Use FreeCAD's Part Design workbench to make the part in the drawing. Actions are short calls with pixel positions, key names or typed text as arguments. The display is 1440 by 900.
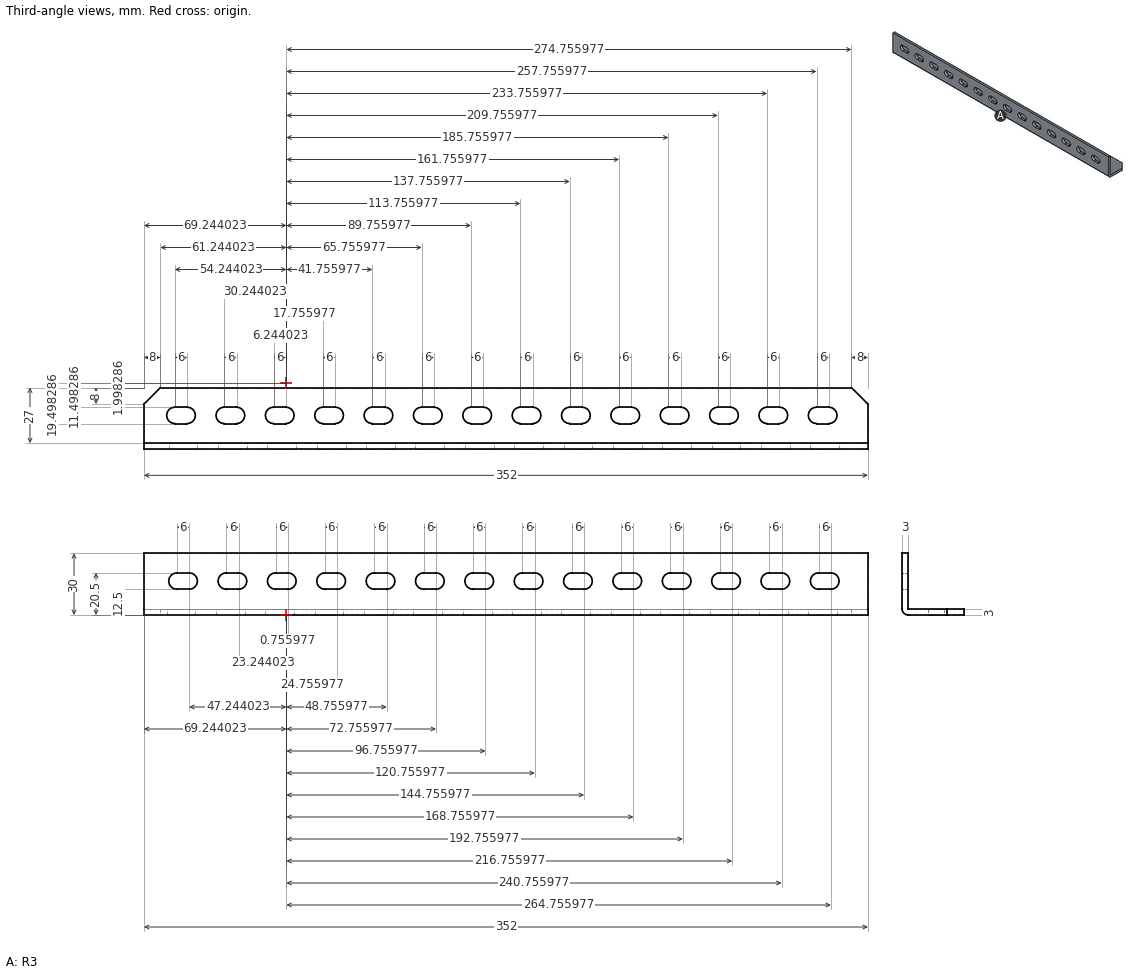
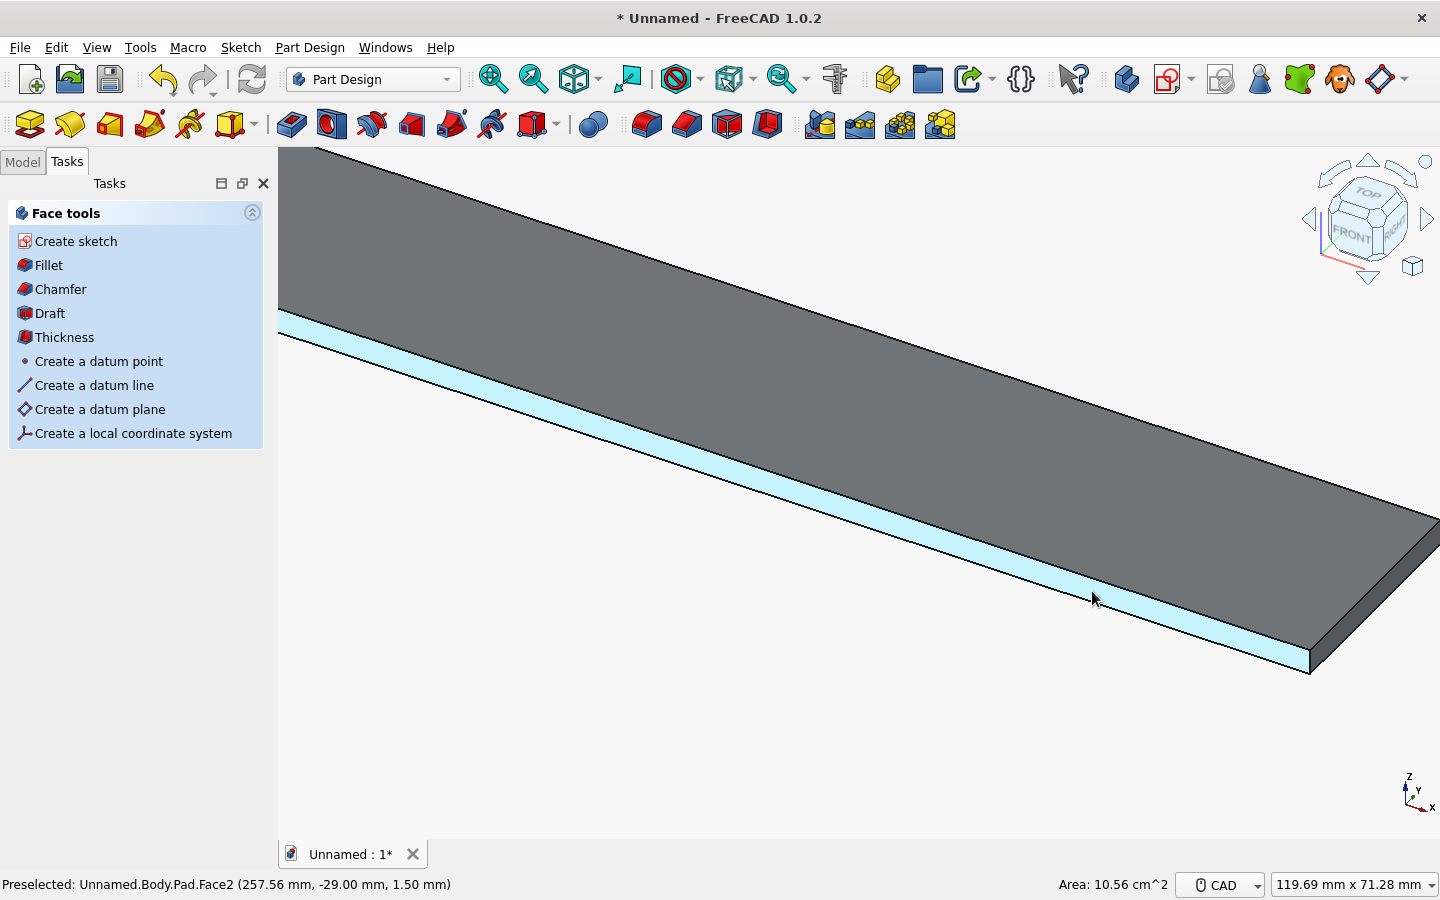
click(1168, 80)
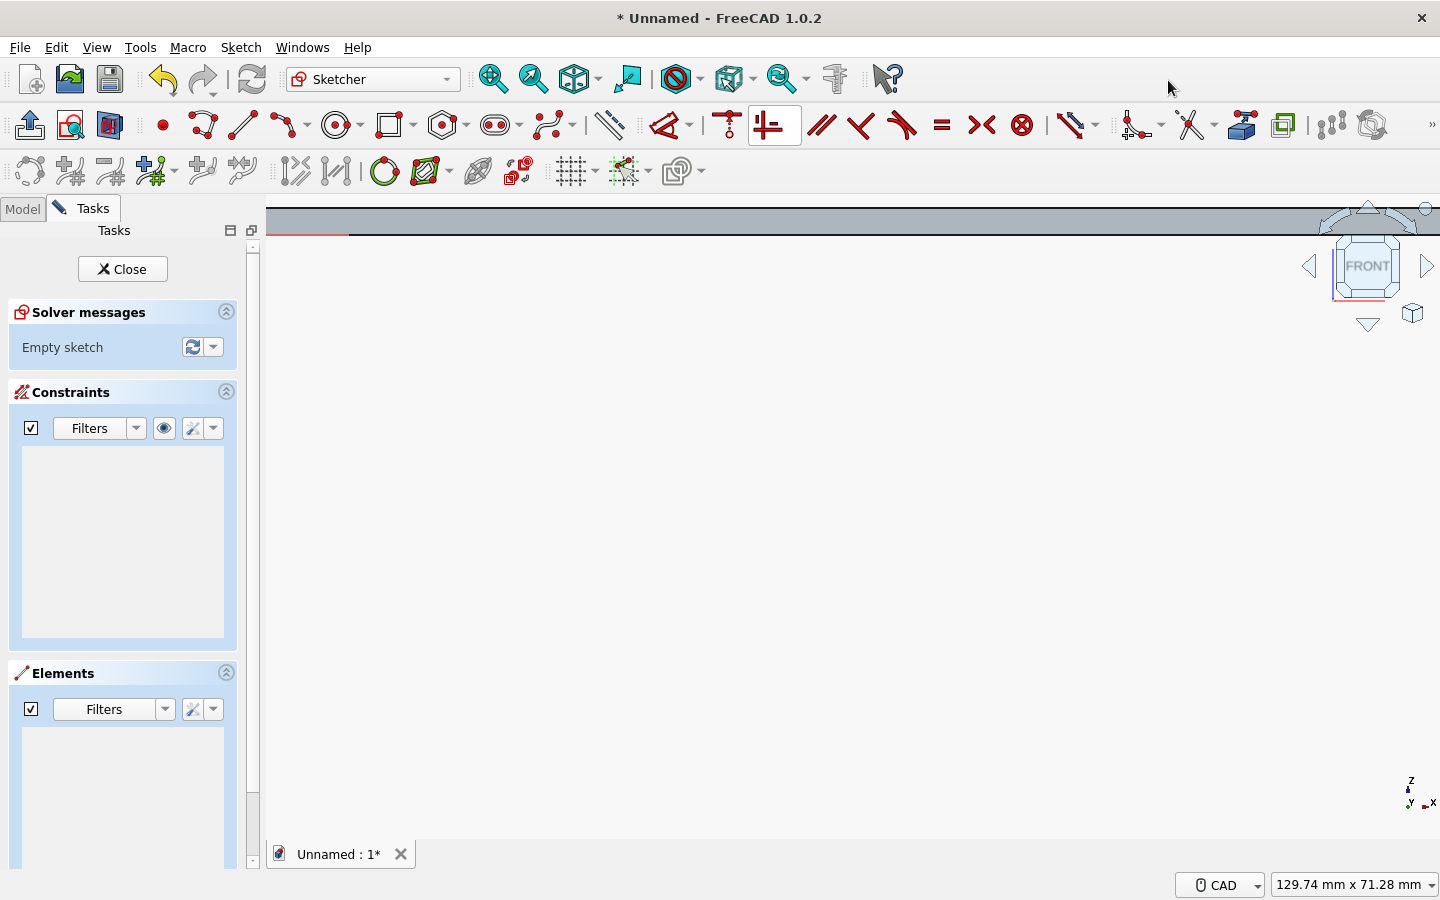
scroll(990, 622, down, 8)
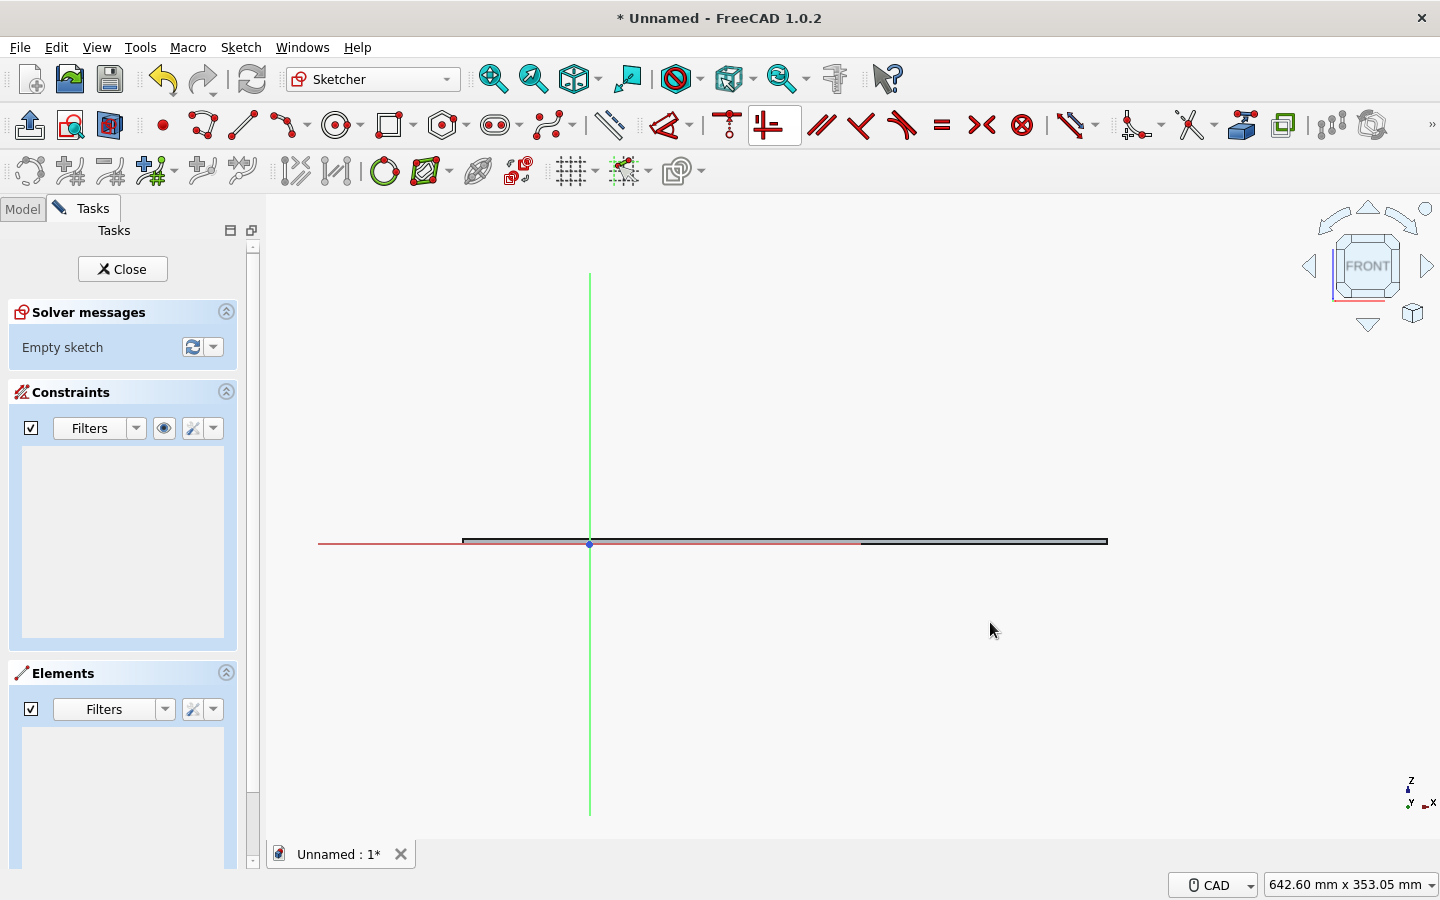
click(390, 126)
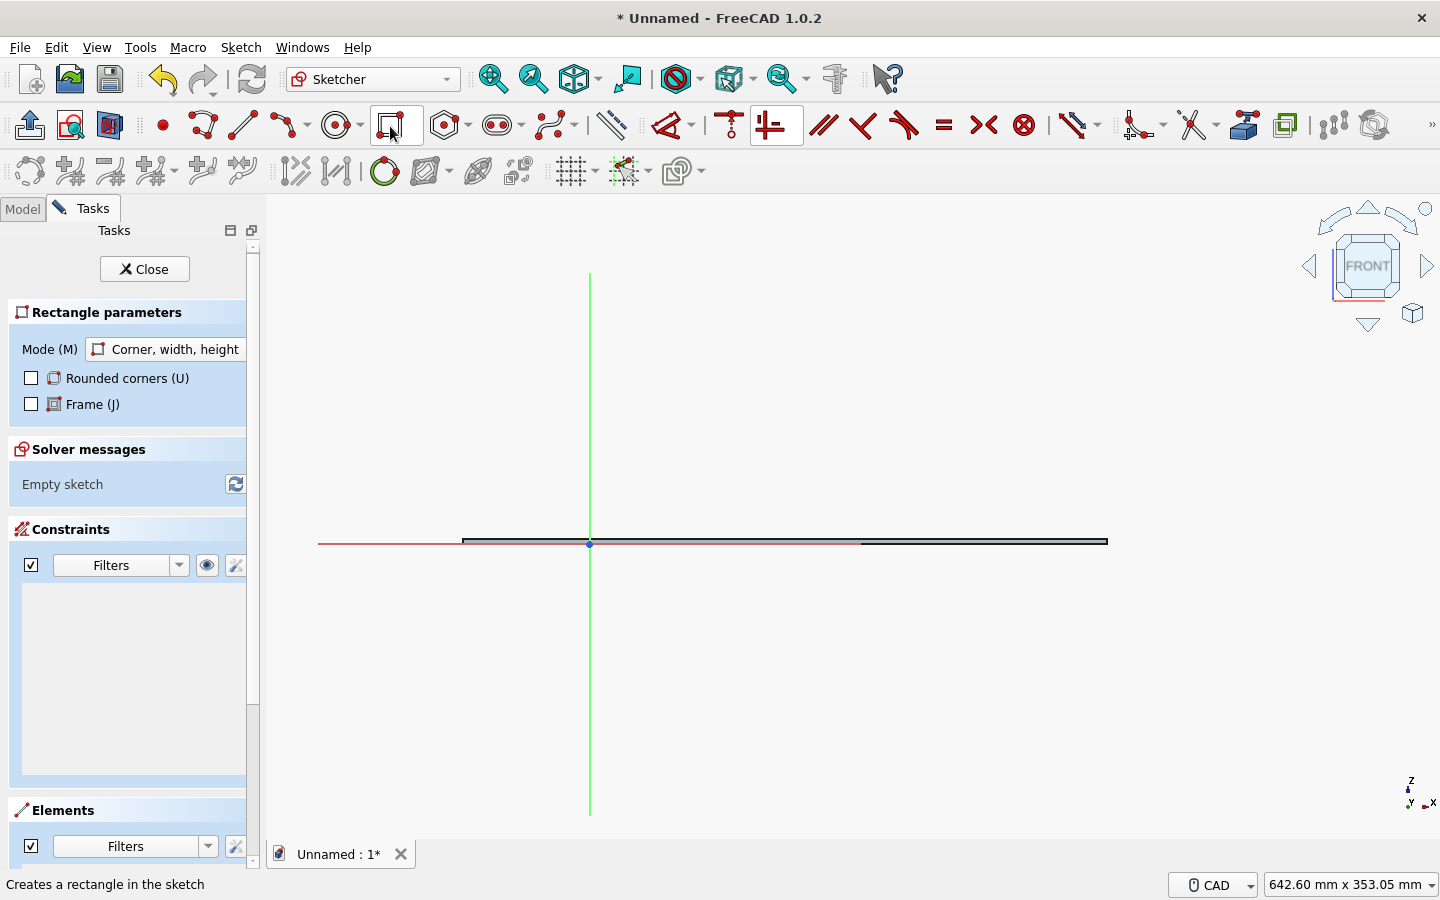
click(463, 490)
click(1107, 544)
key(Escape)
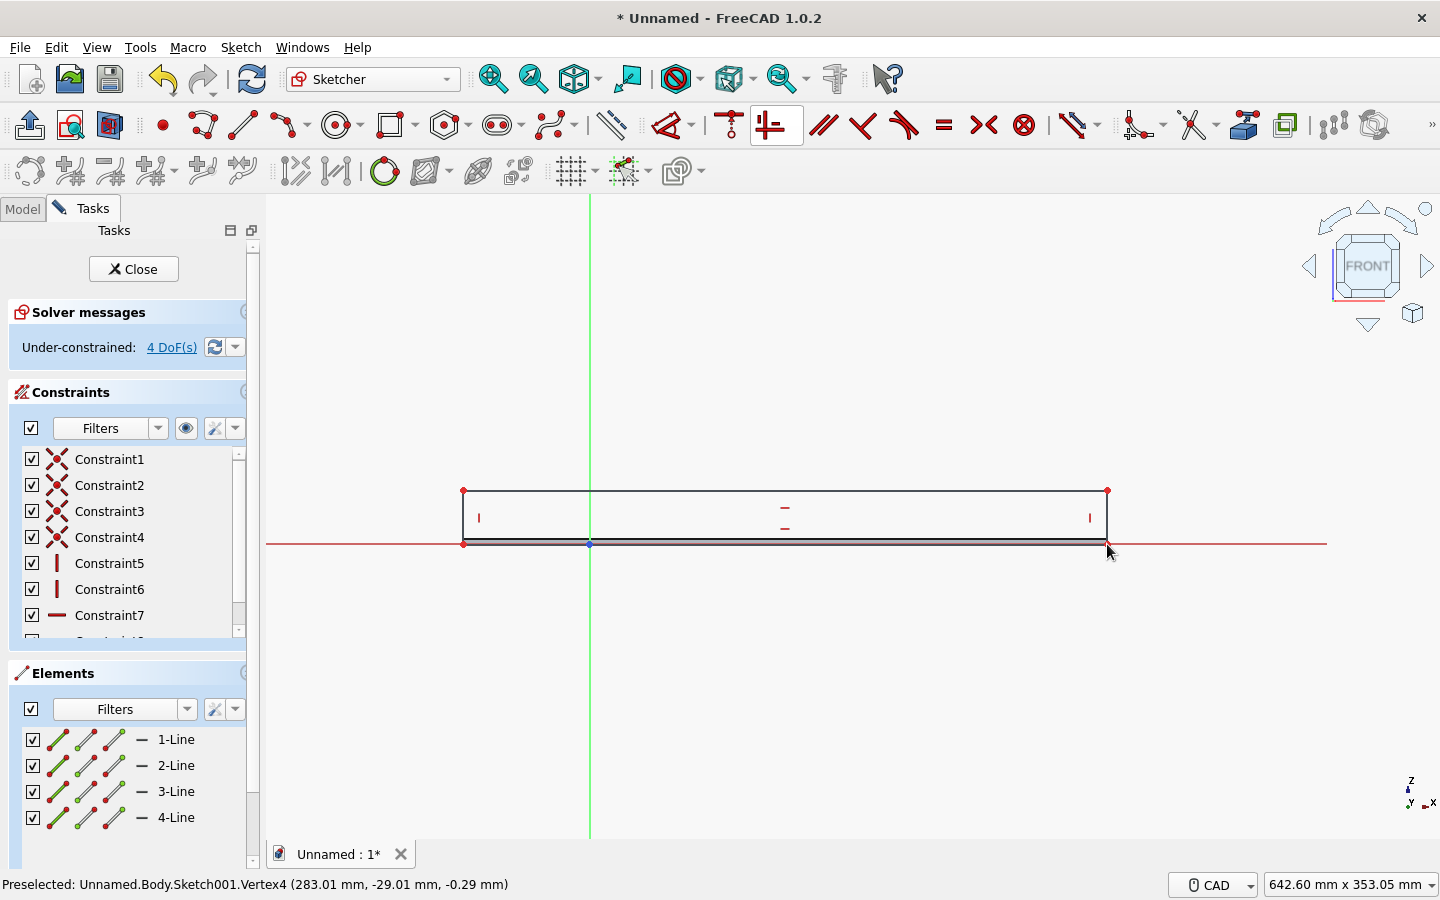
click(463, 545)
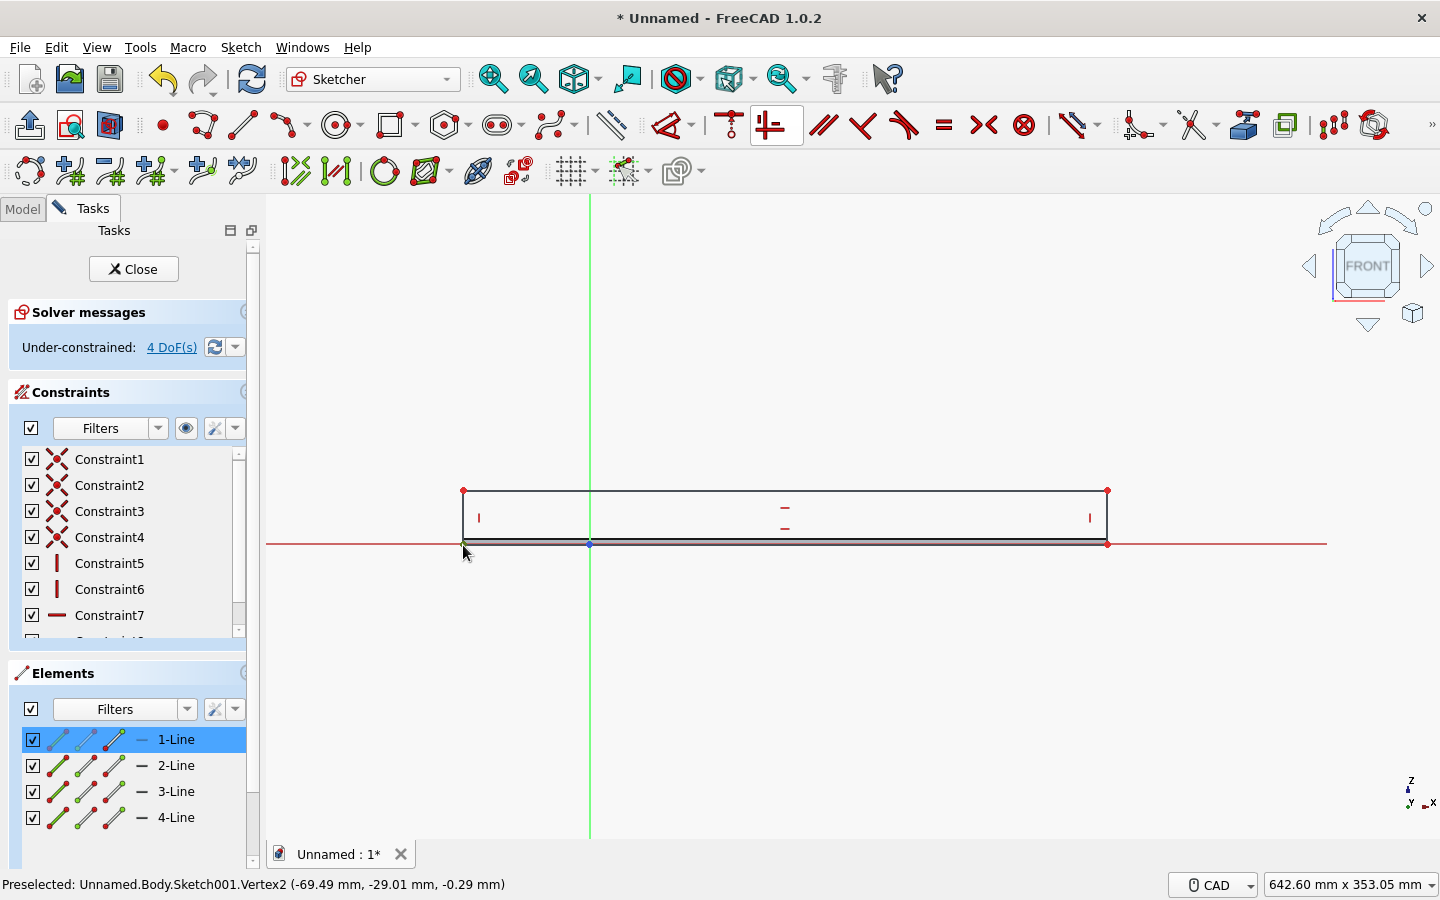
click(364, 544)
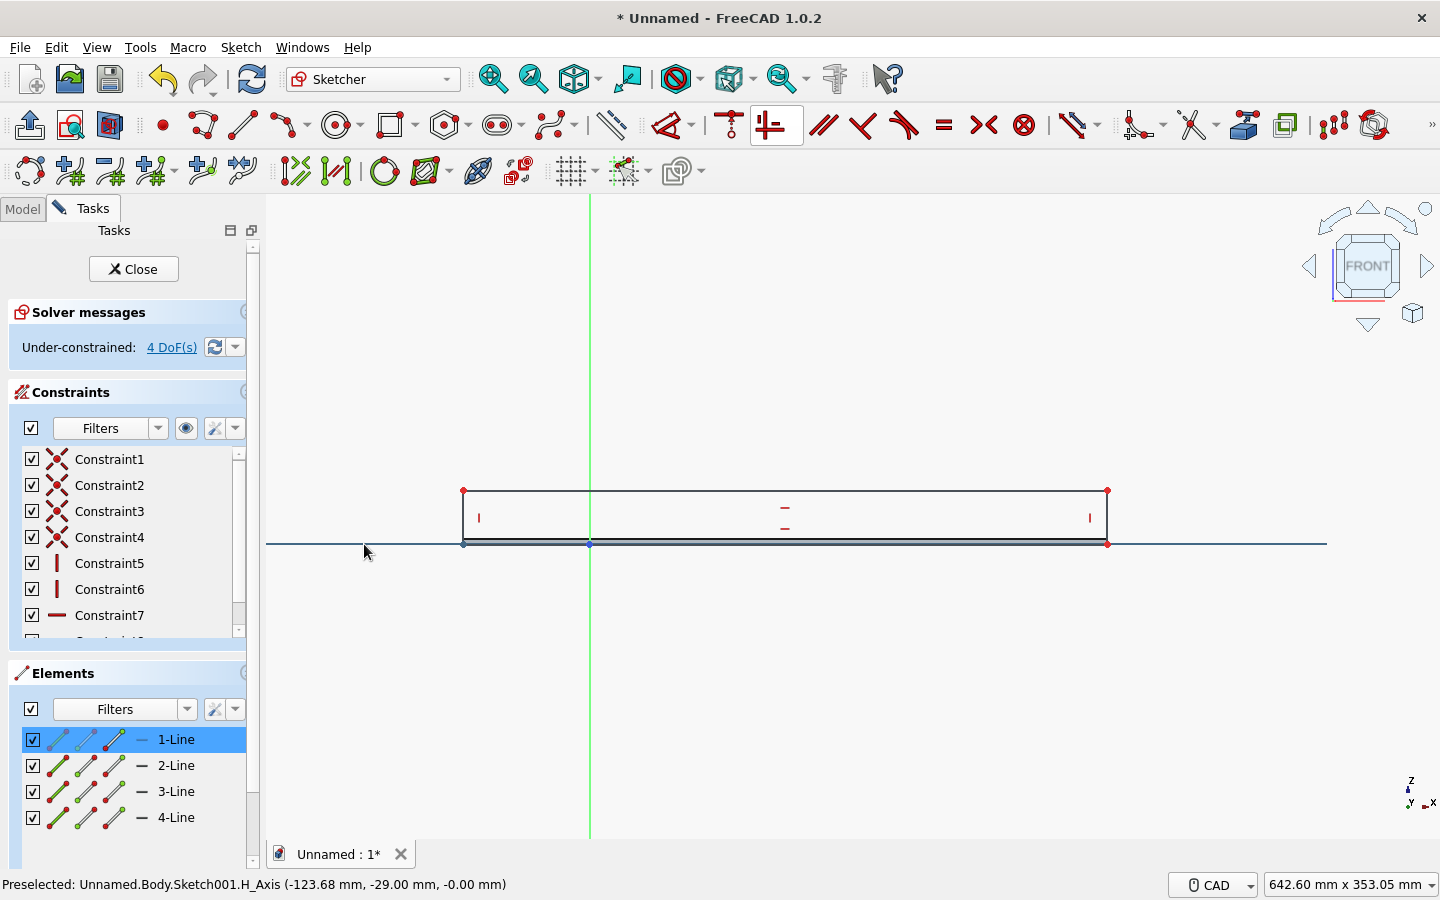
click(730, 126)